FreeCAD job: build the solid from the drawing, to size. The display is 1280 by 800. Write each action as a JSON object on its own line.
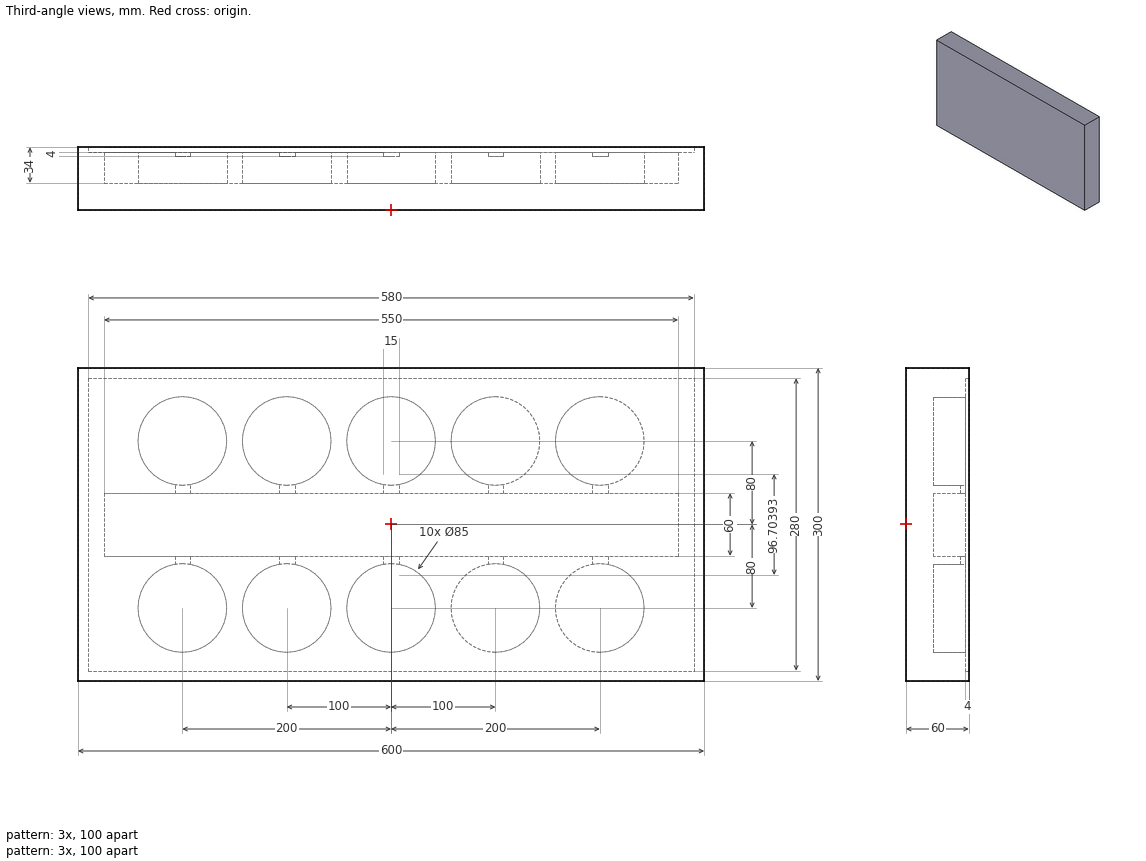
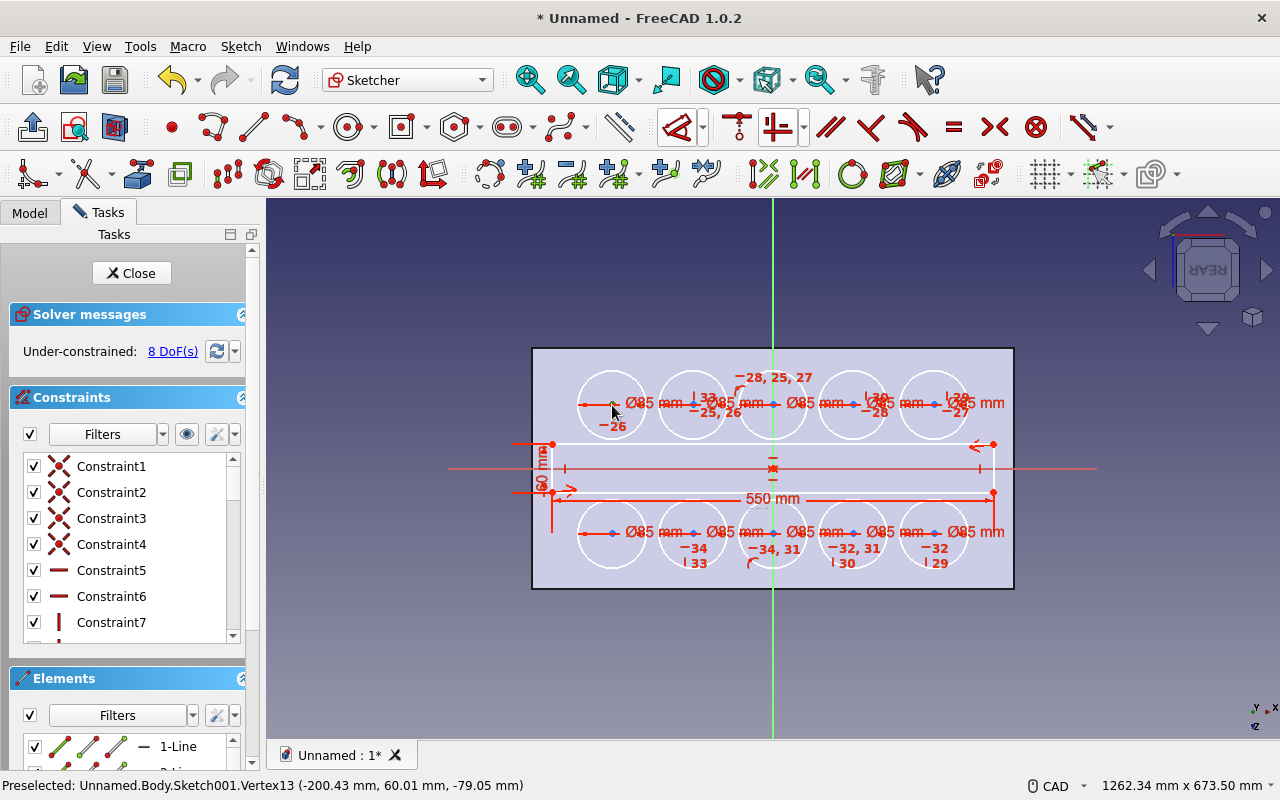
{"action": "left_click", "coordinate": [612, 534]}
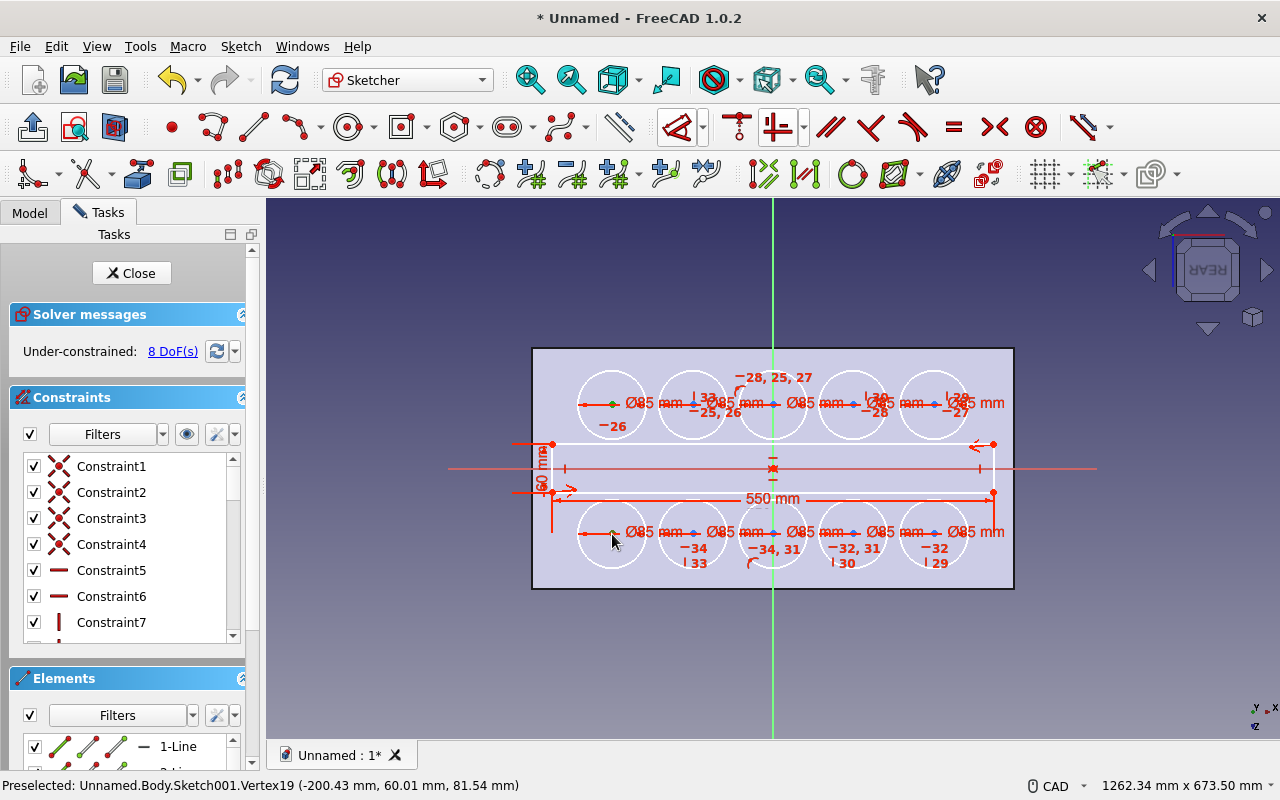
{"action": "key", "text": "v"}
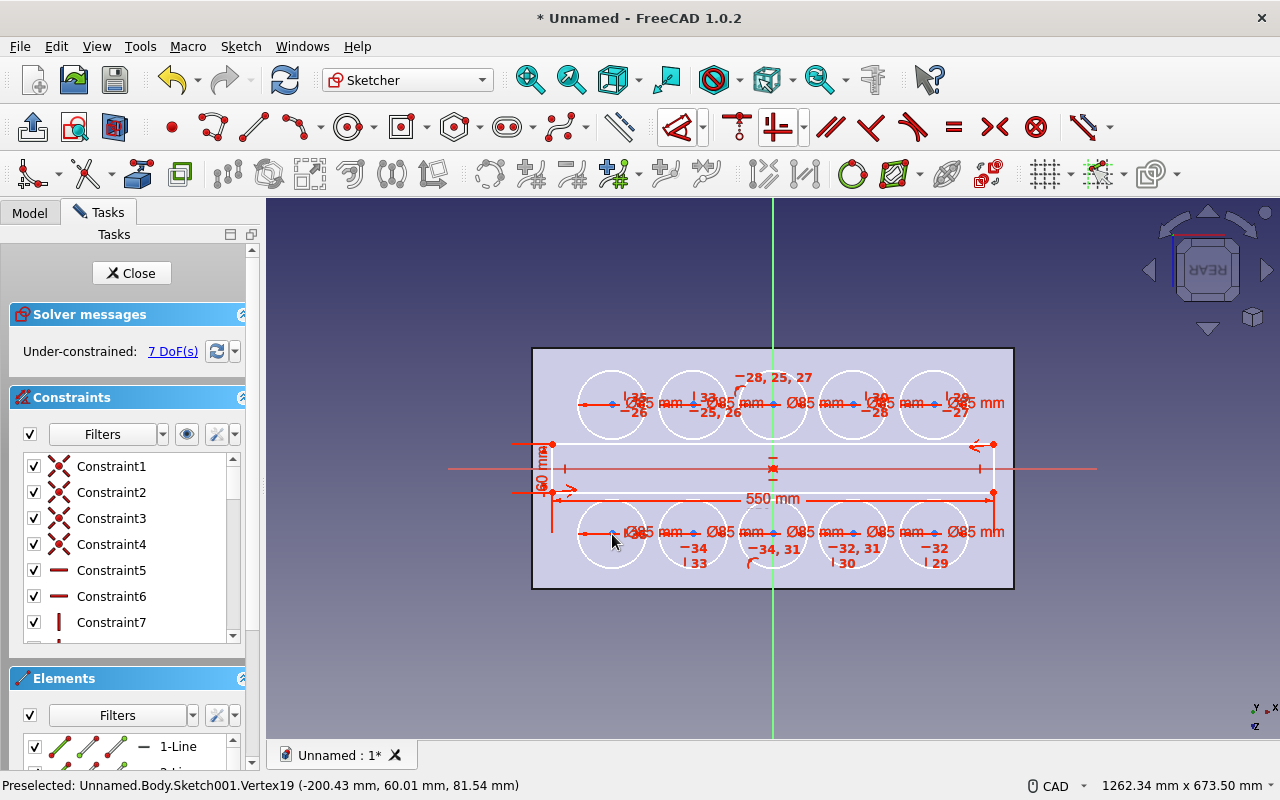
{"action": "left_click", "coordinate": [693, 534]}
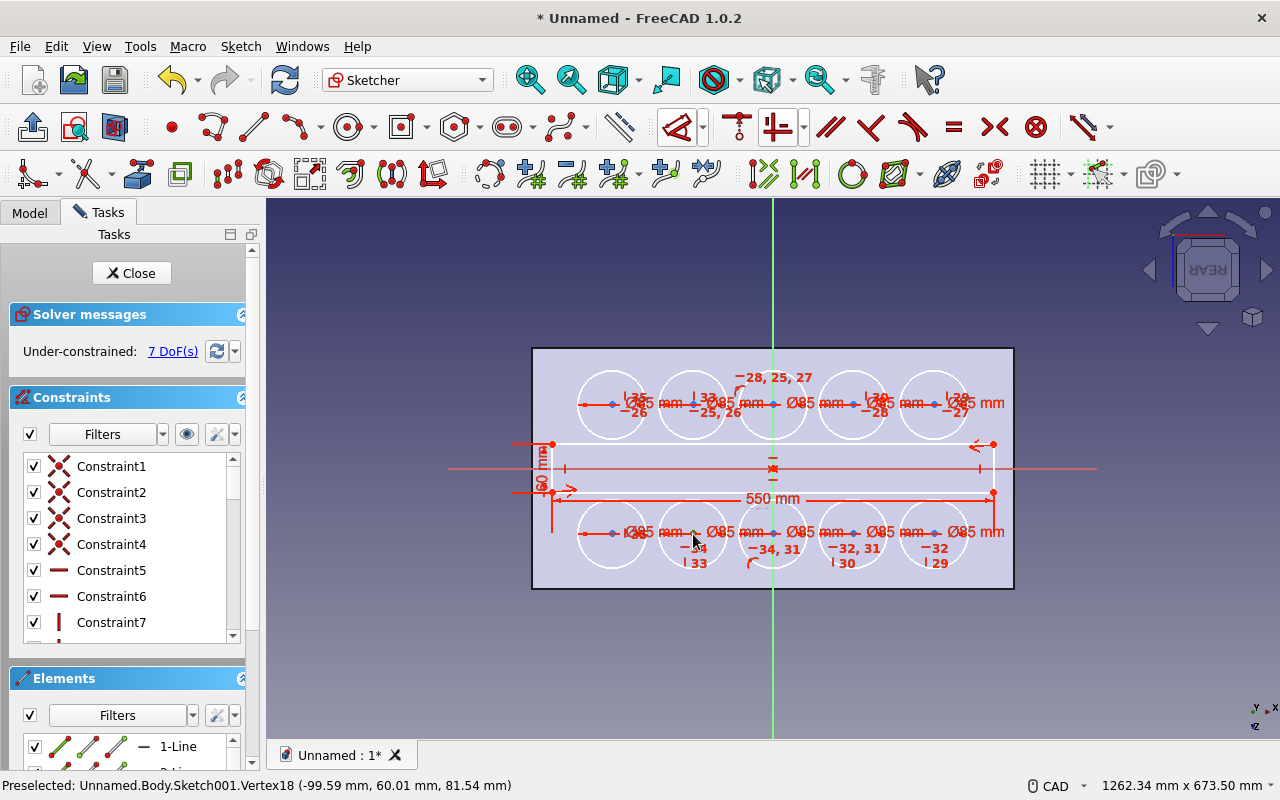
{"action": "left_click", "coordinate": [612, 534]}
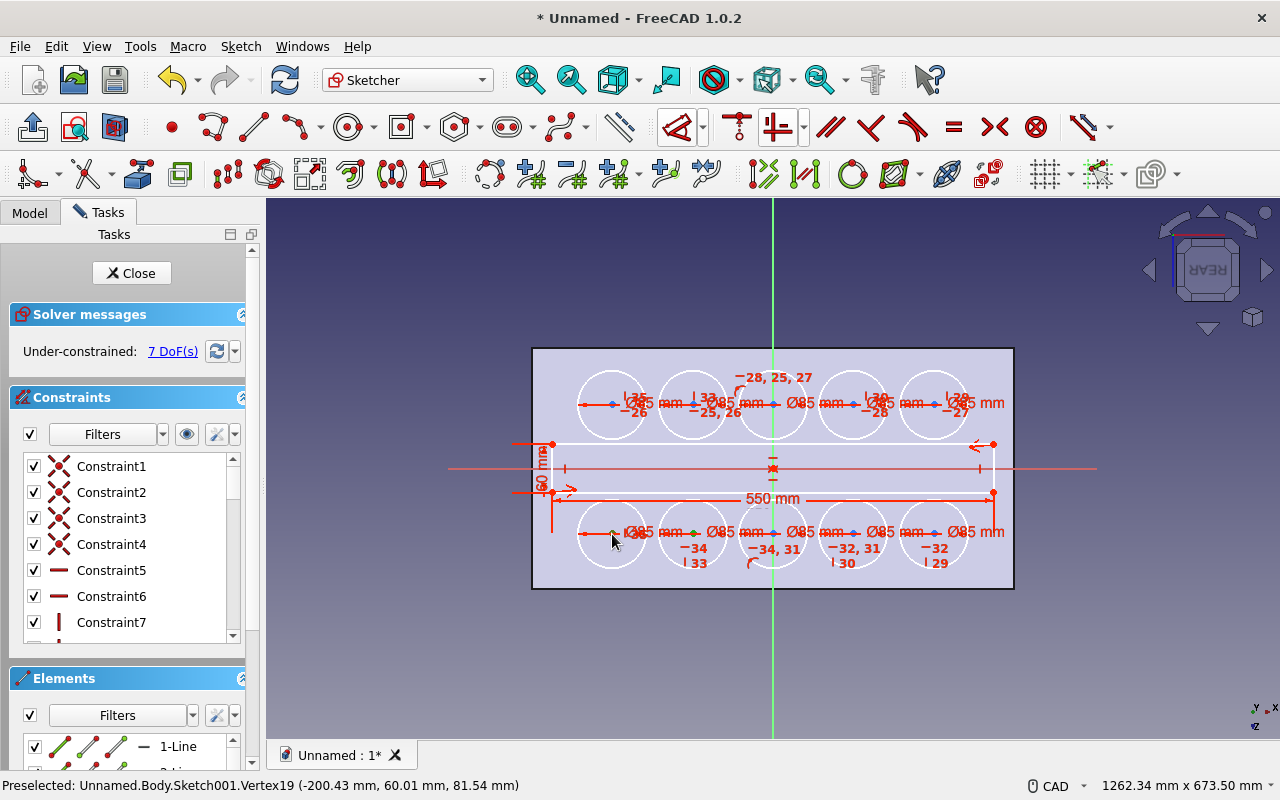
{"action": "key", "text": "h"}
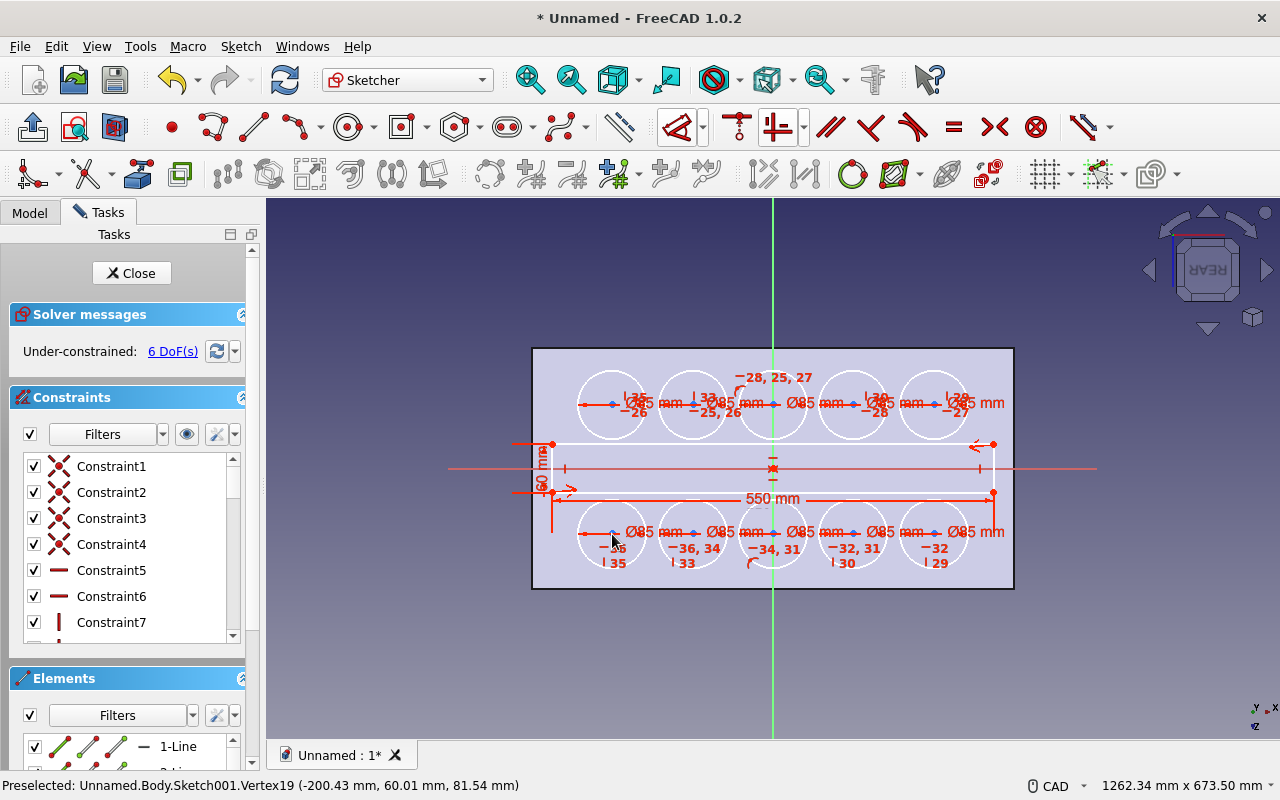
{"action": "key", "text": "d"}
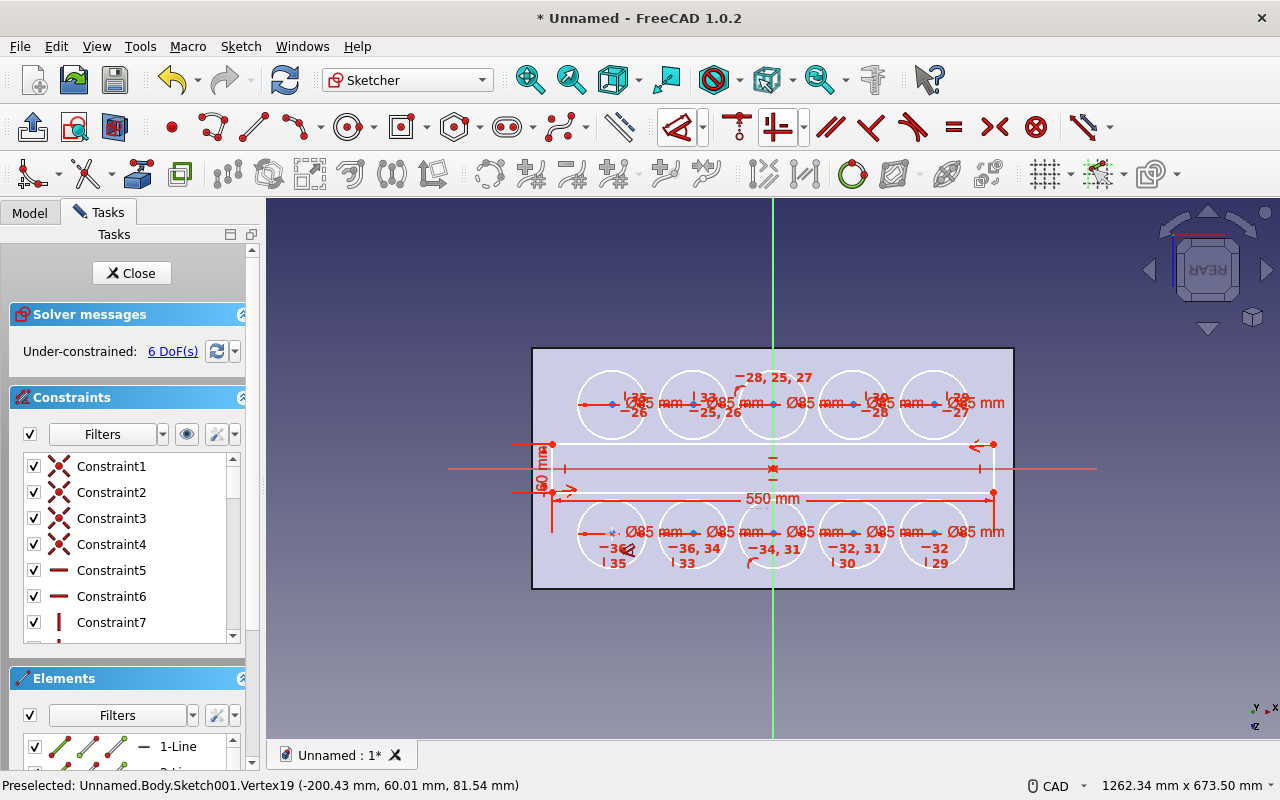
{"action": "left_click", "coordinate": [773, 405]}
{"action": "left_click", "coordinate": [855, 422]}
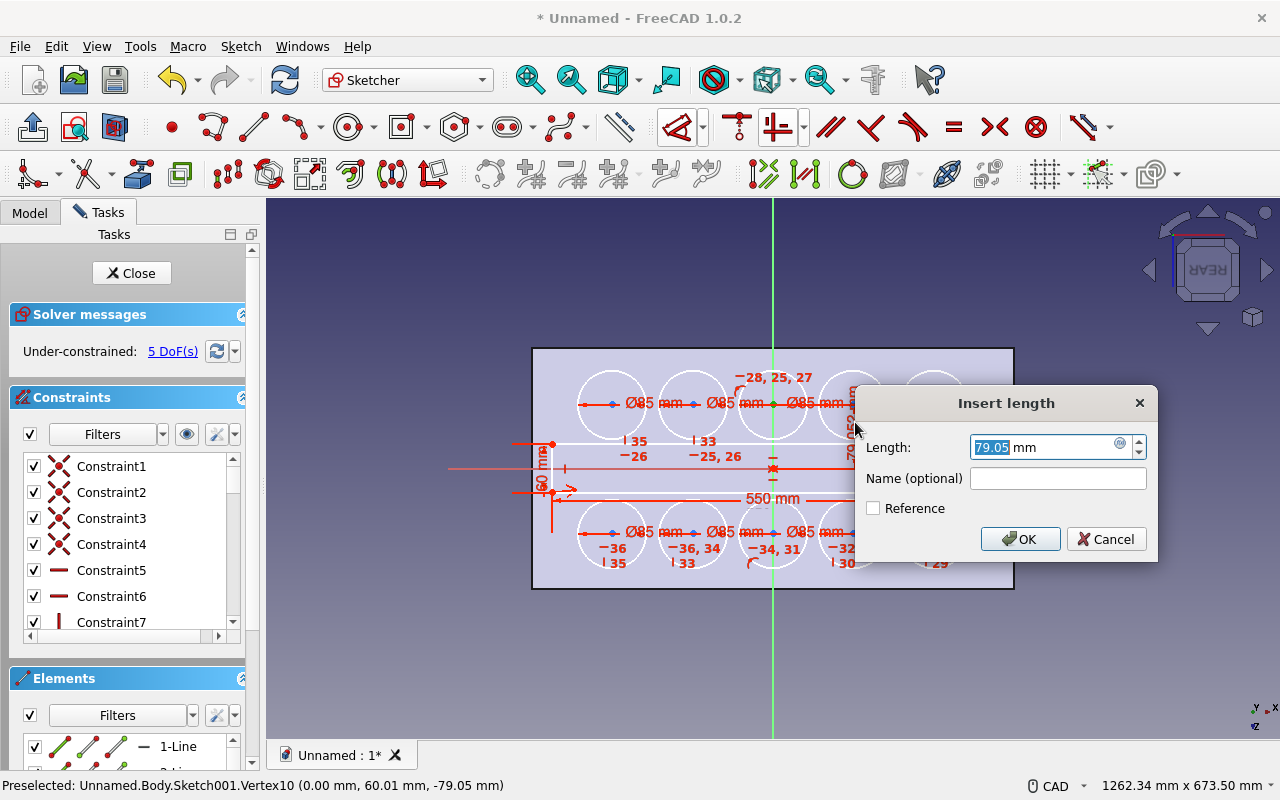
{"action": "type", "text": "80"}
{"action": "key", "text": "Return"}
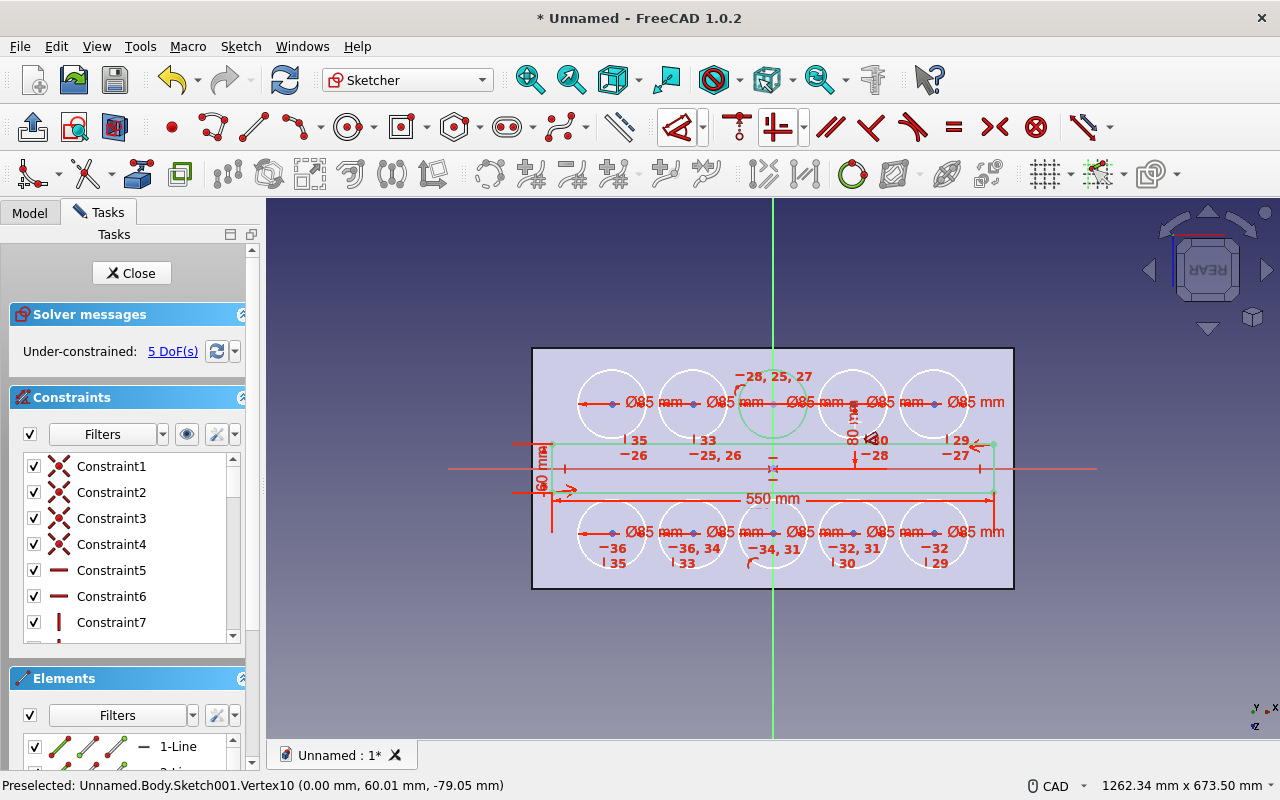
{"action": "left_click", "coordinate": [773, 534]}
{"action": "left_click", "coordinate": [855, 516]}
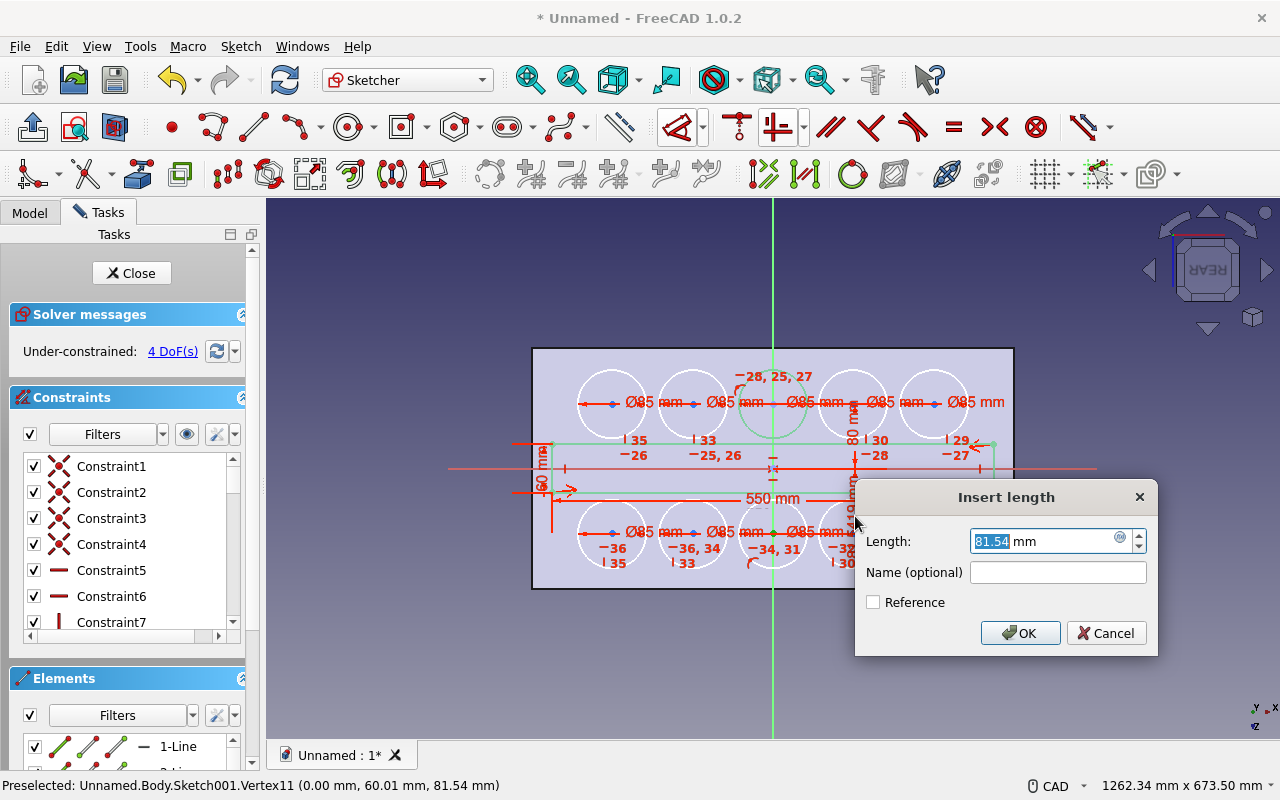
{"action": "type", "text": "80"}
{"action": "key", "text": "Return"}